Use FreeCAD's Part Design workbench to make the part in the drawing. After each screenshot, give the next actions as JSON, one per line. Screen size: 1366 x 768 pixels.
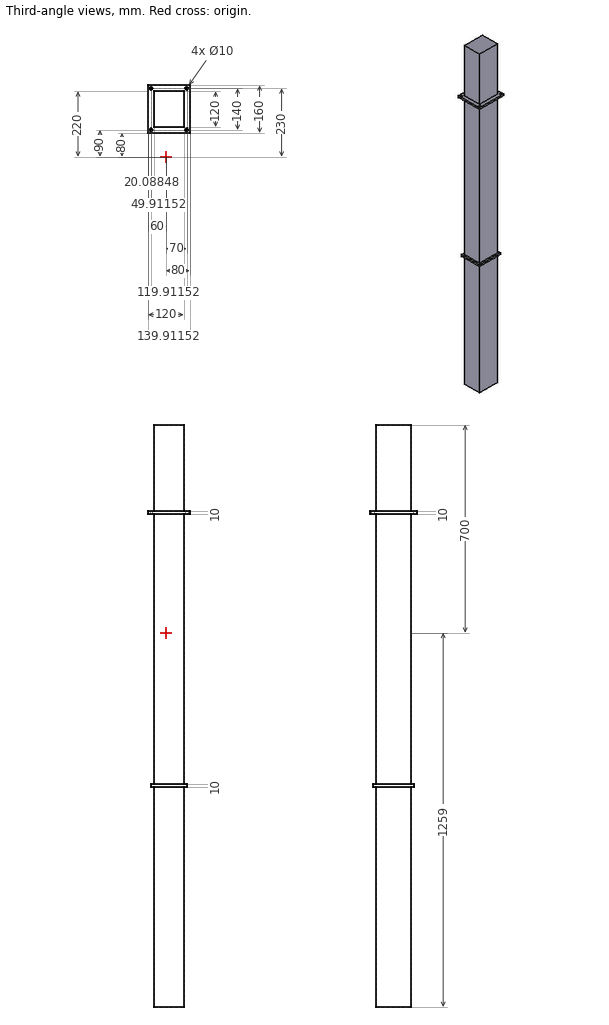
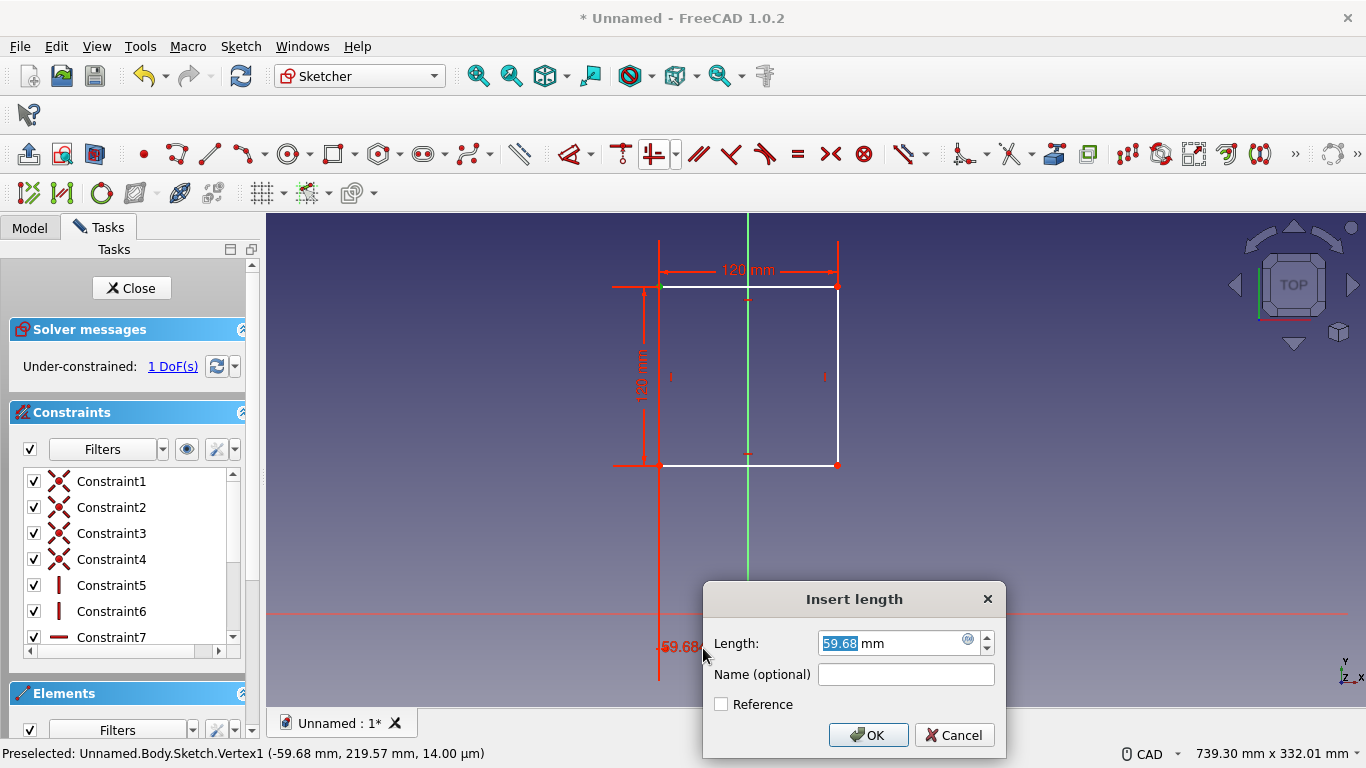
{"action": "type", "text": "60"}
{"action": "key", "text": "Return"}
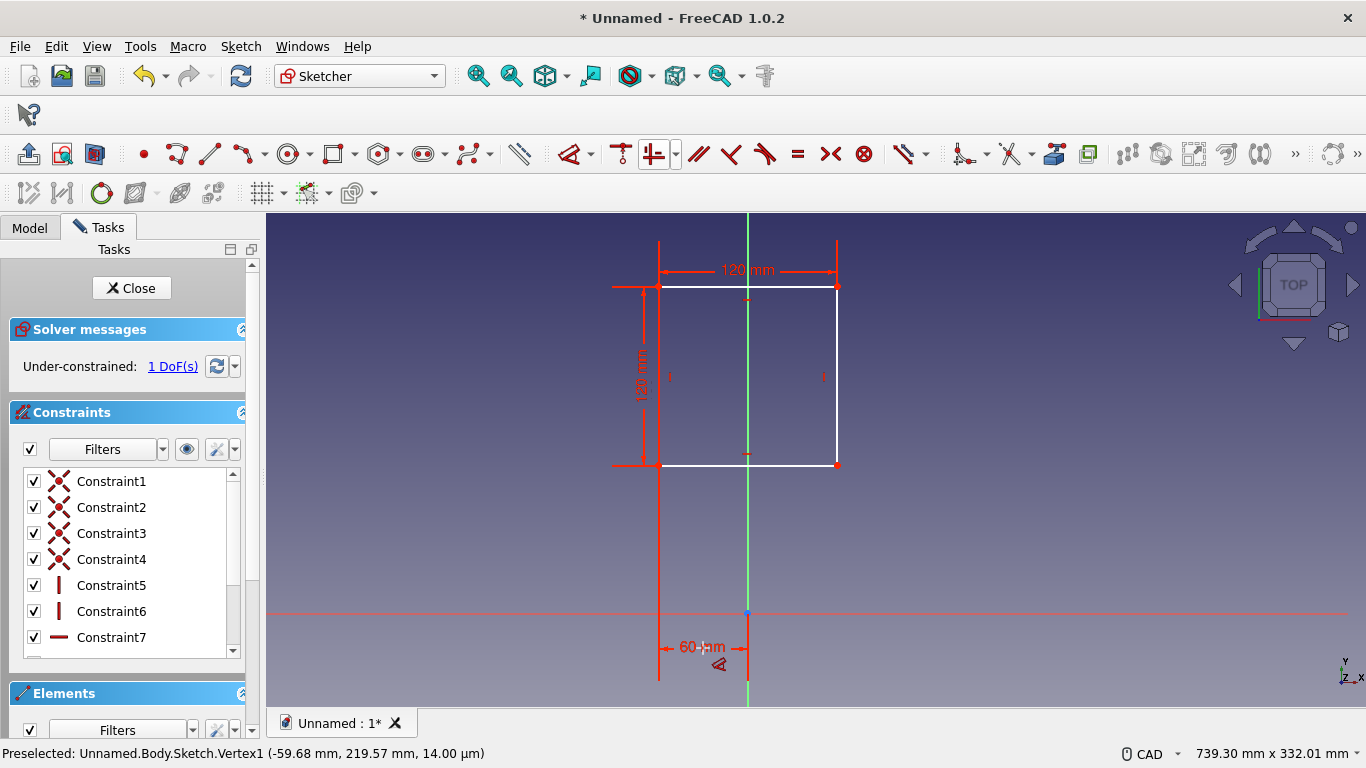
{"action": "left_click", "coordinate": [659, 287]}
{"action": "left_click", "coordinate": [625, 450]}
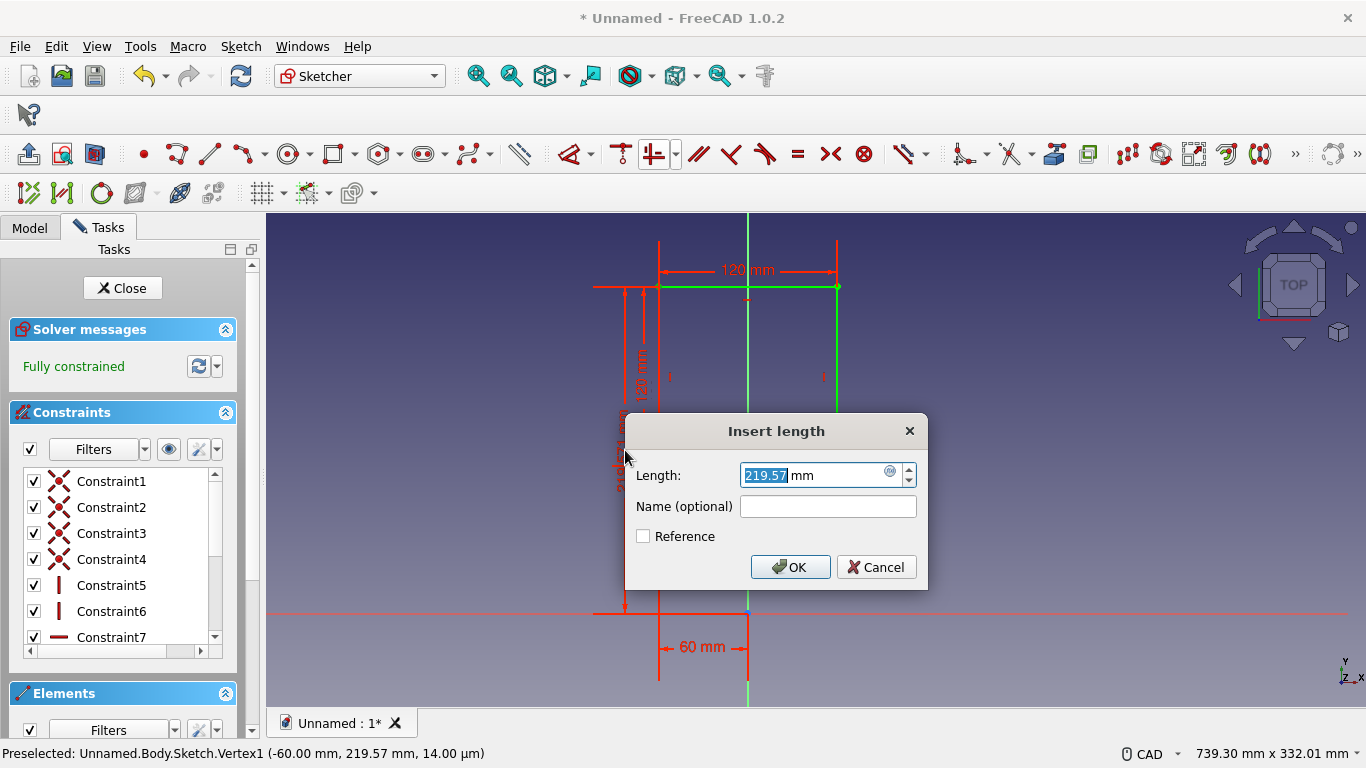
{"action": "type", "text": "220"}
{"action": "key", "text": "Return"}
{"action": "key", "text": "Escape"}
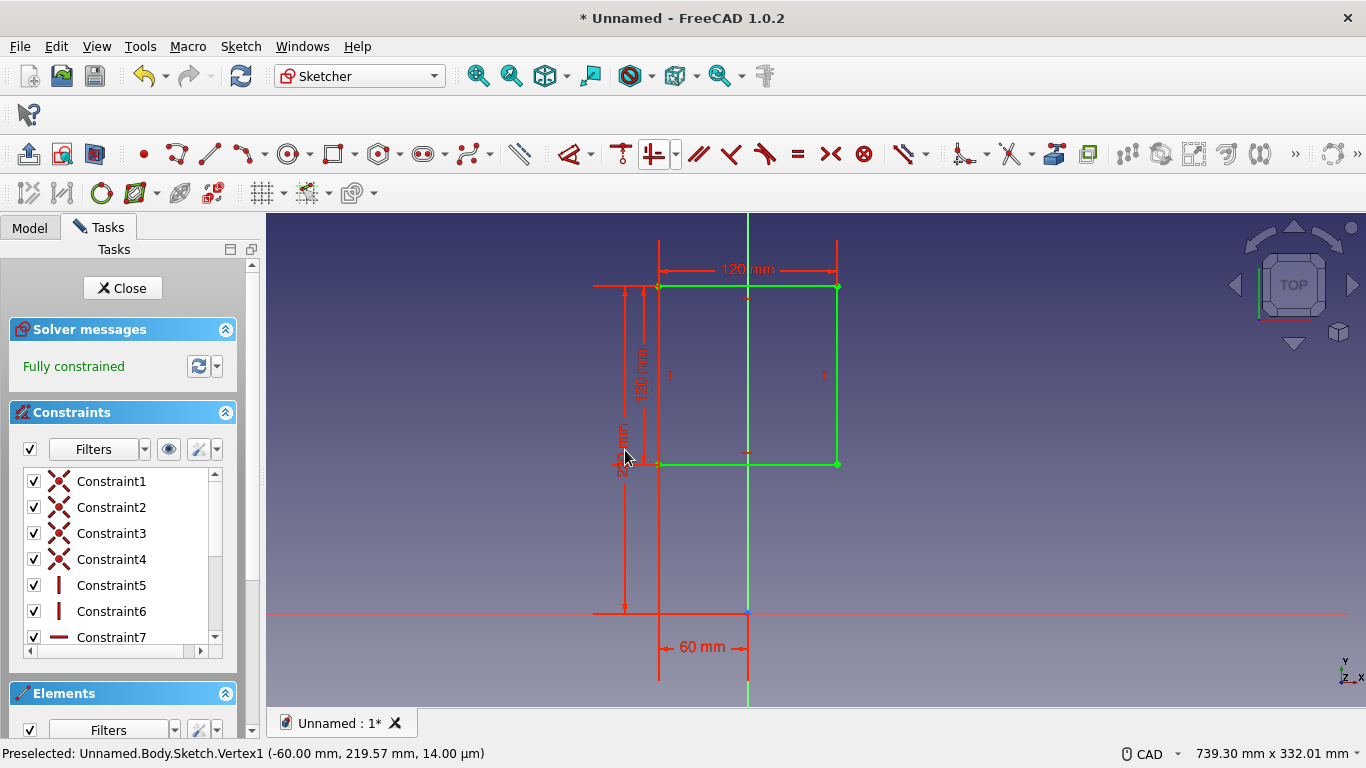
{"action": "left_click", "coordinate": [123, 288]}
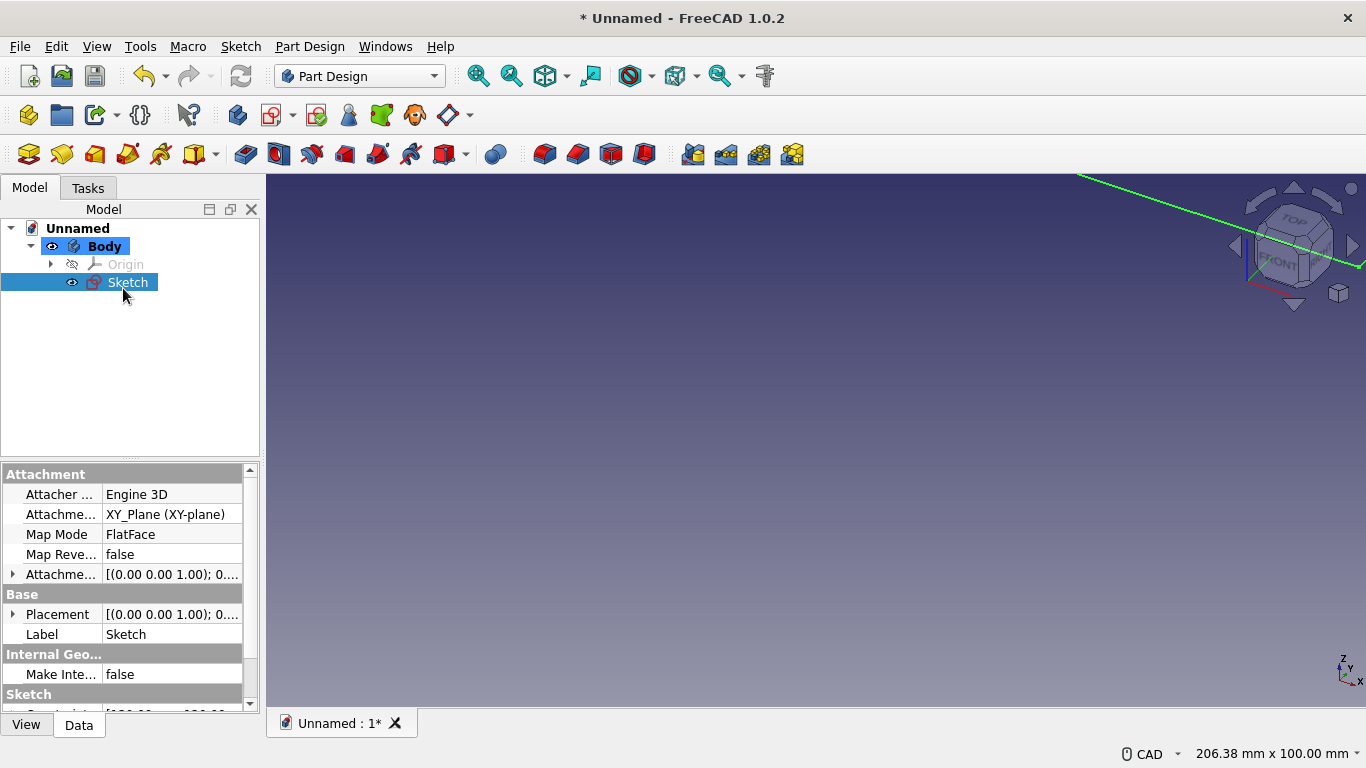
{"action": "left_click", "coordinate": [29, 154]}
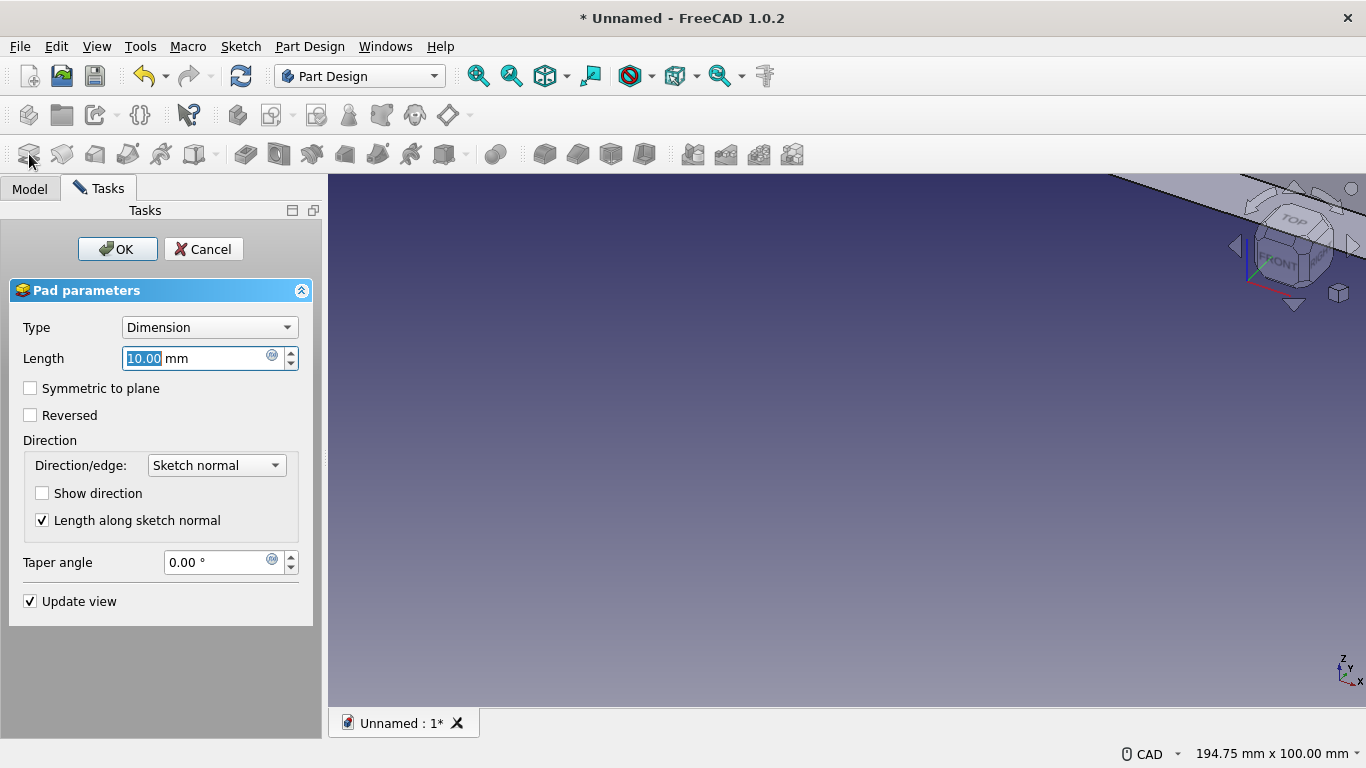
{"action": "left_click", "coordinate": [210, 328]}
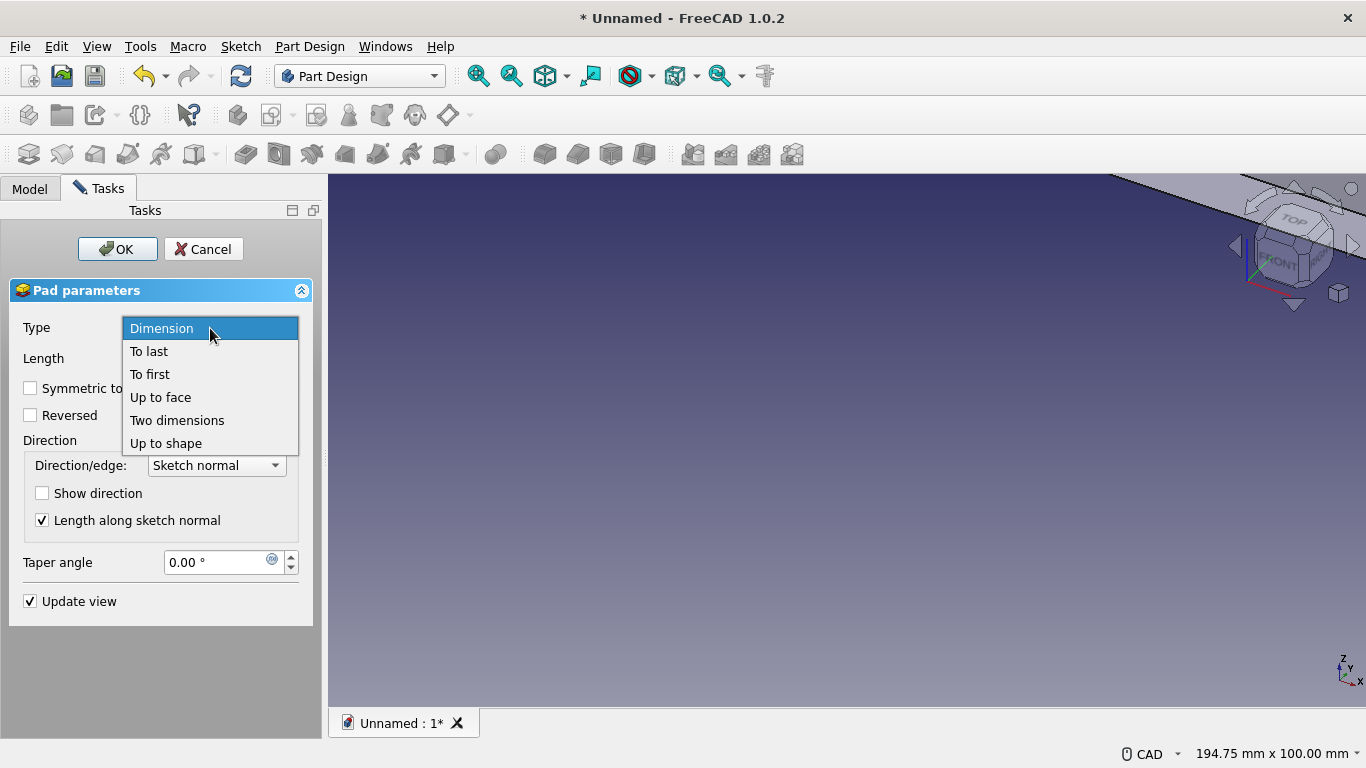
{"action": "left_click", "coordinate": [208, 420]}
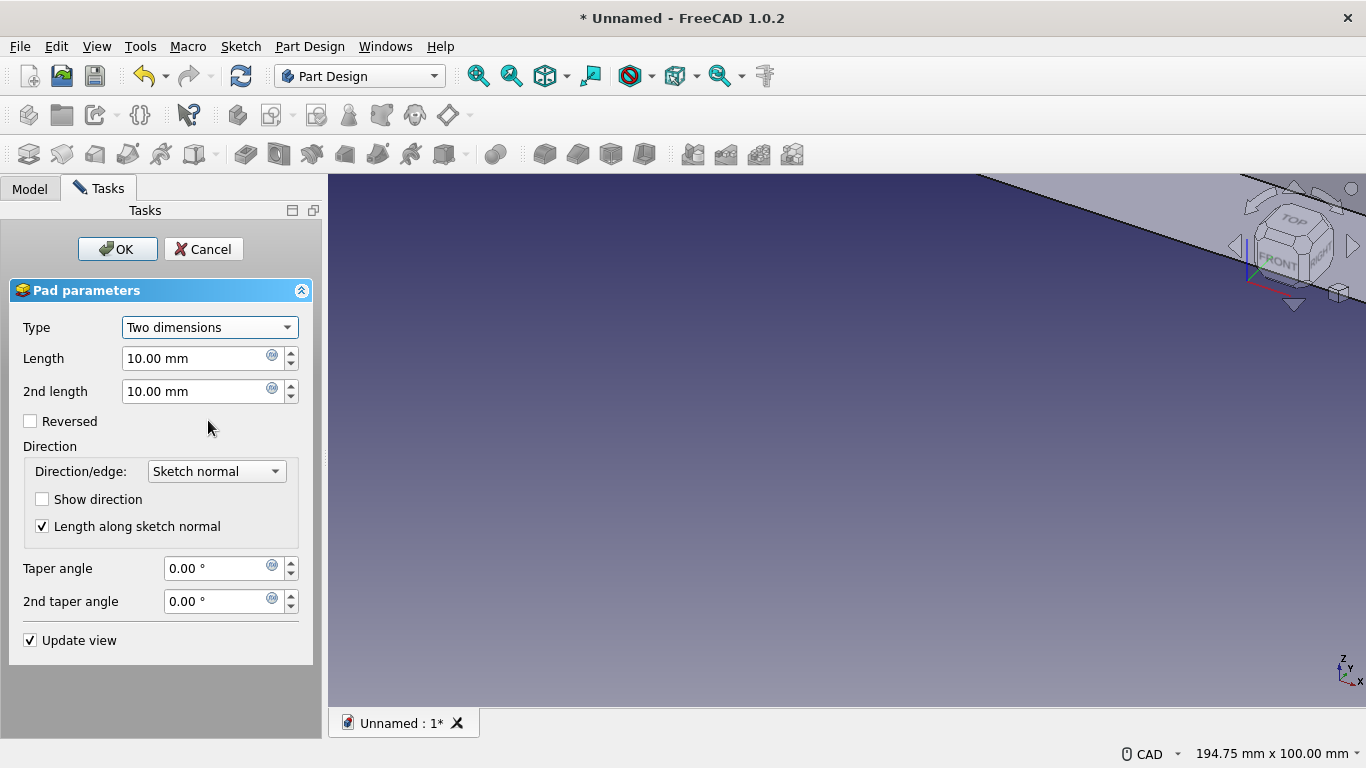
{"action": "triple_click", "coordinate": [204, 358]}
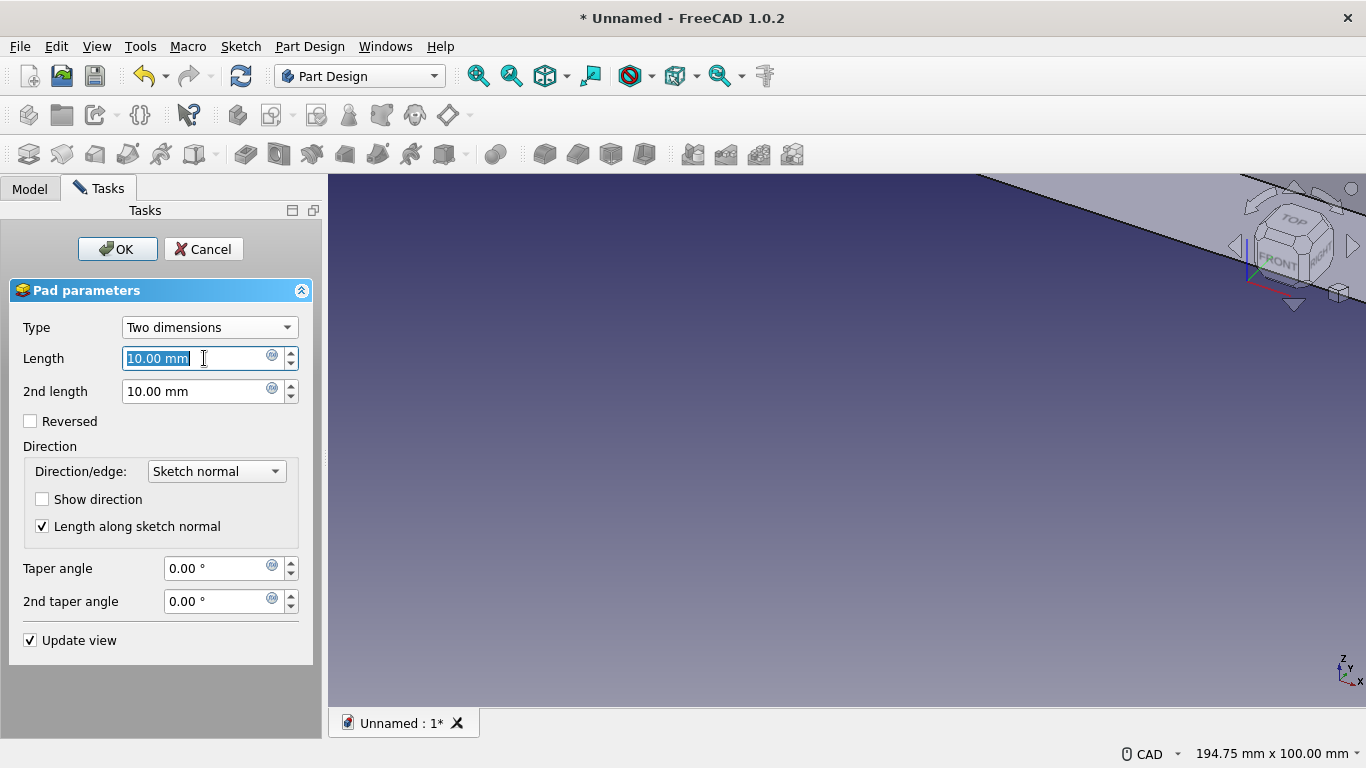
{"action": "type", "text": "700"}
{"action": "key", "text": "Tab"}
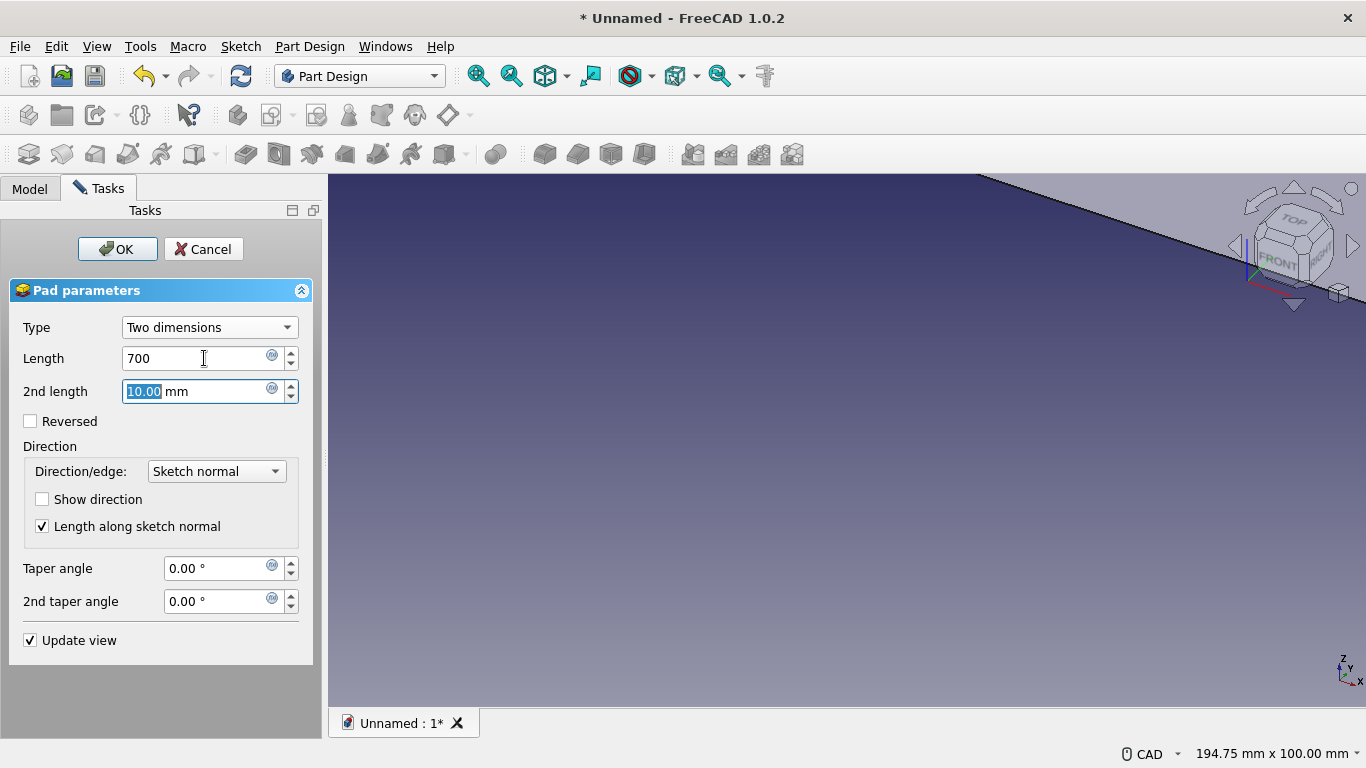
{"action": "type", "text": "1259"}
{"action": "key", "text": "Tab"}